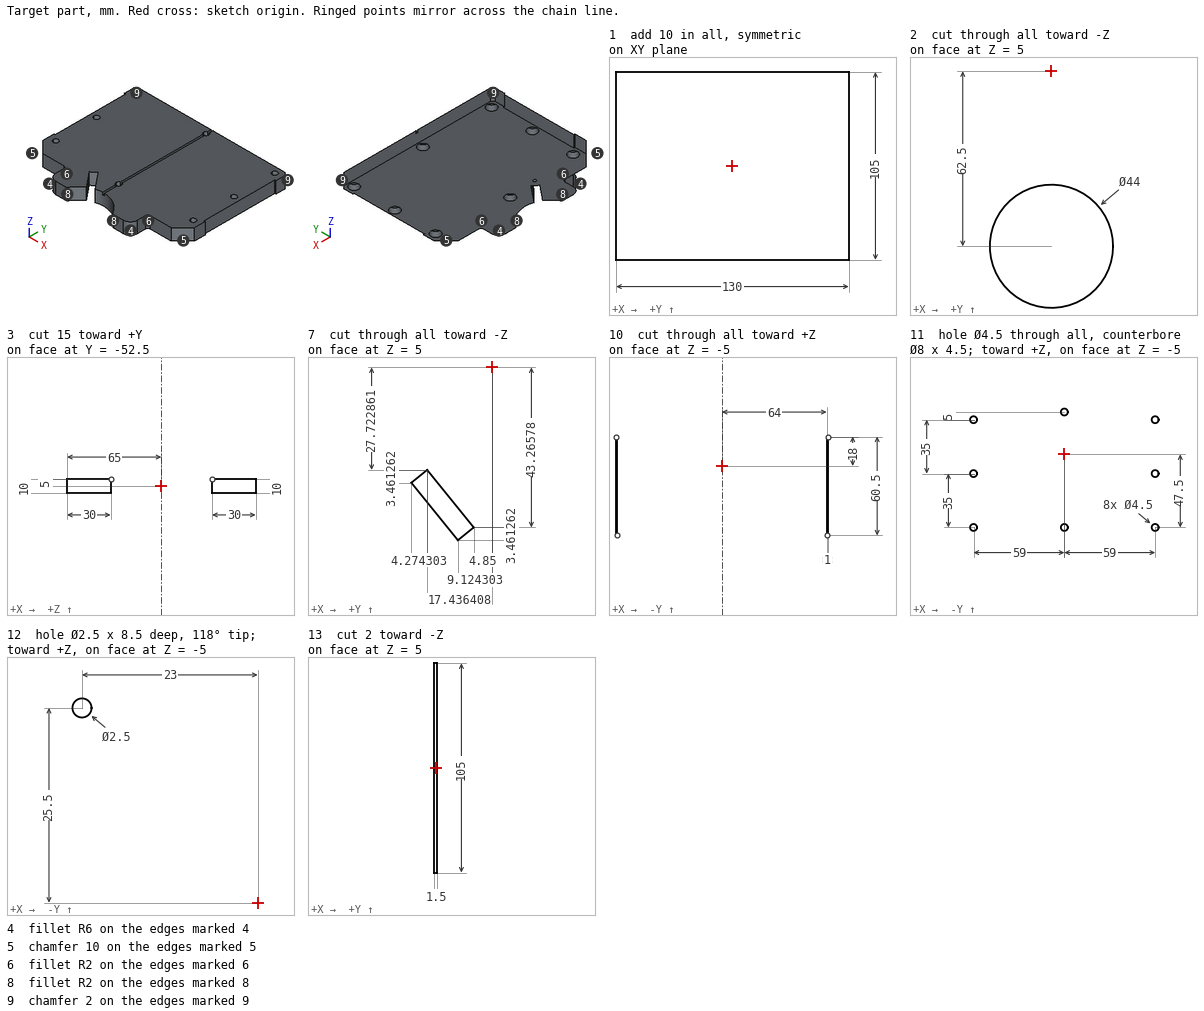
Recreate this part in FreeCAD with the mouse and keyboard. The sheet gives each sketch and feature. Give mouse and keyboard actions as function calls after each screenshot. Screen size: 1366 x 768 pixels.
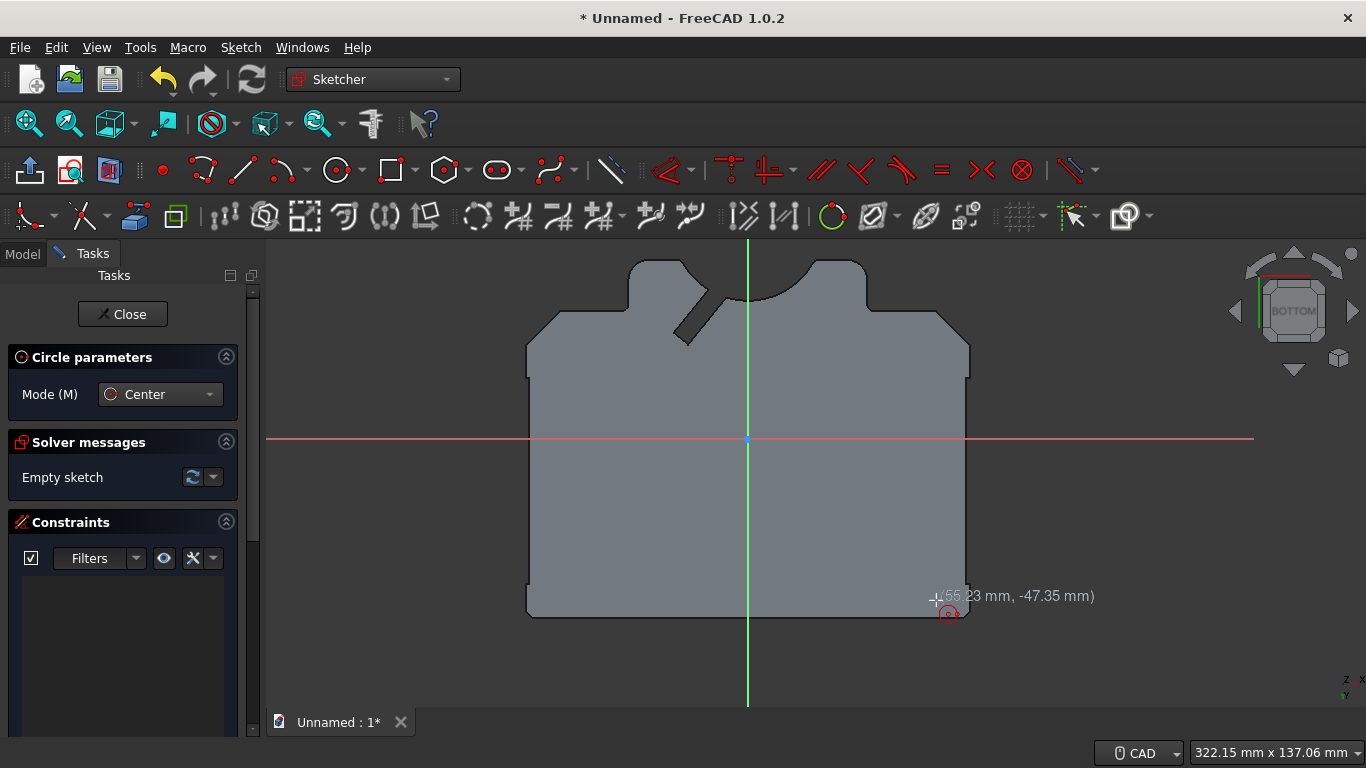
click(949, 601)
move(955, 596)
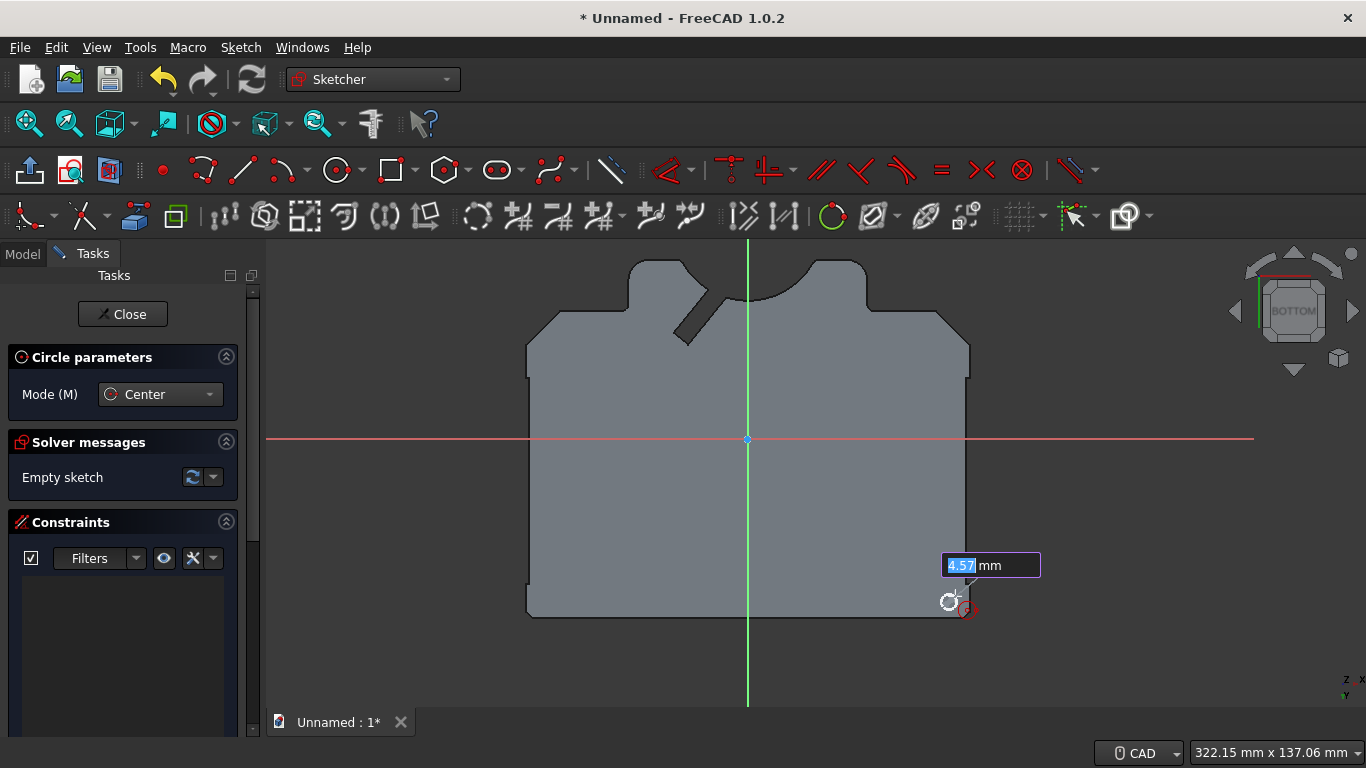
text(4.5)
key(Return)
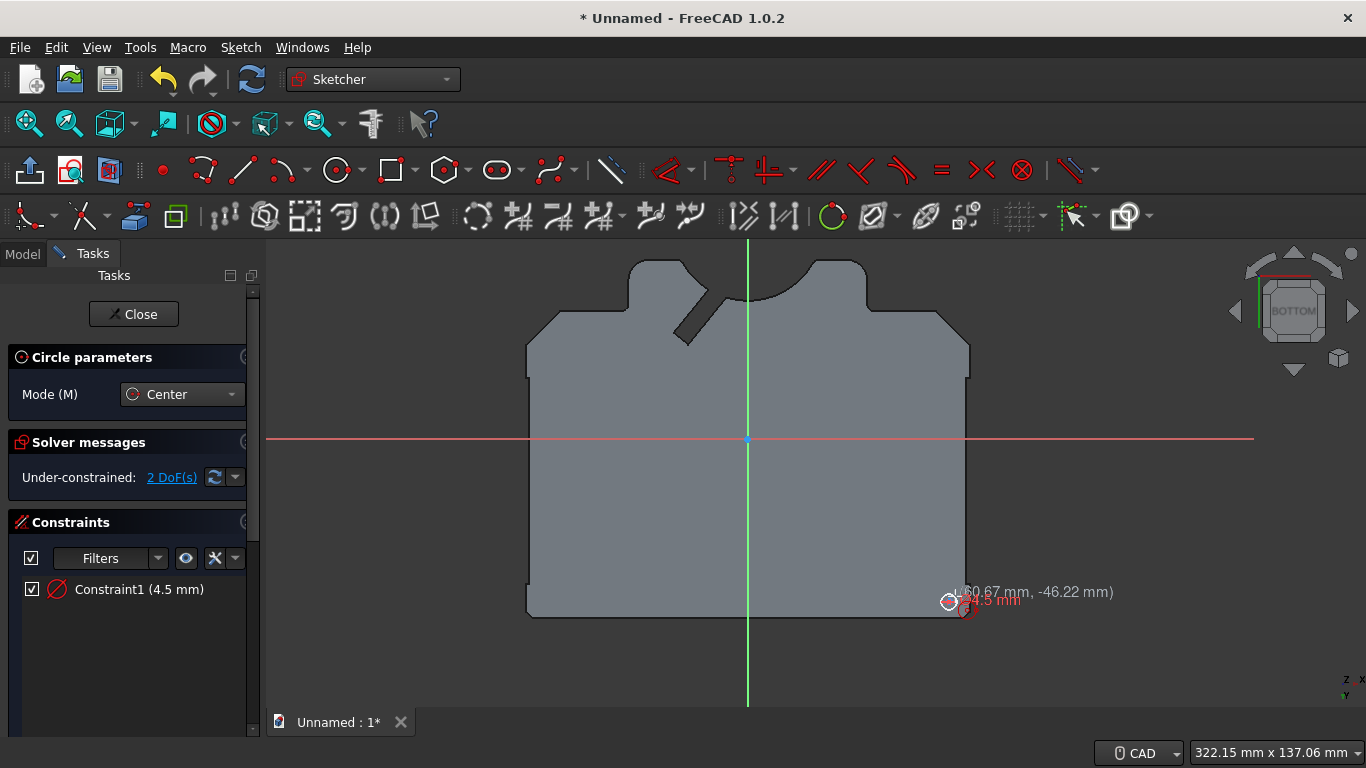
scroll(748, 601, up, 6)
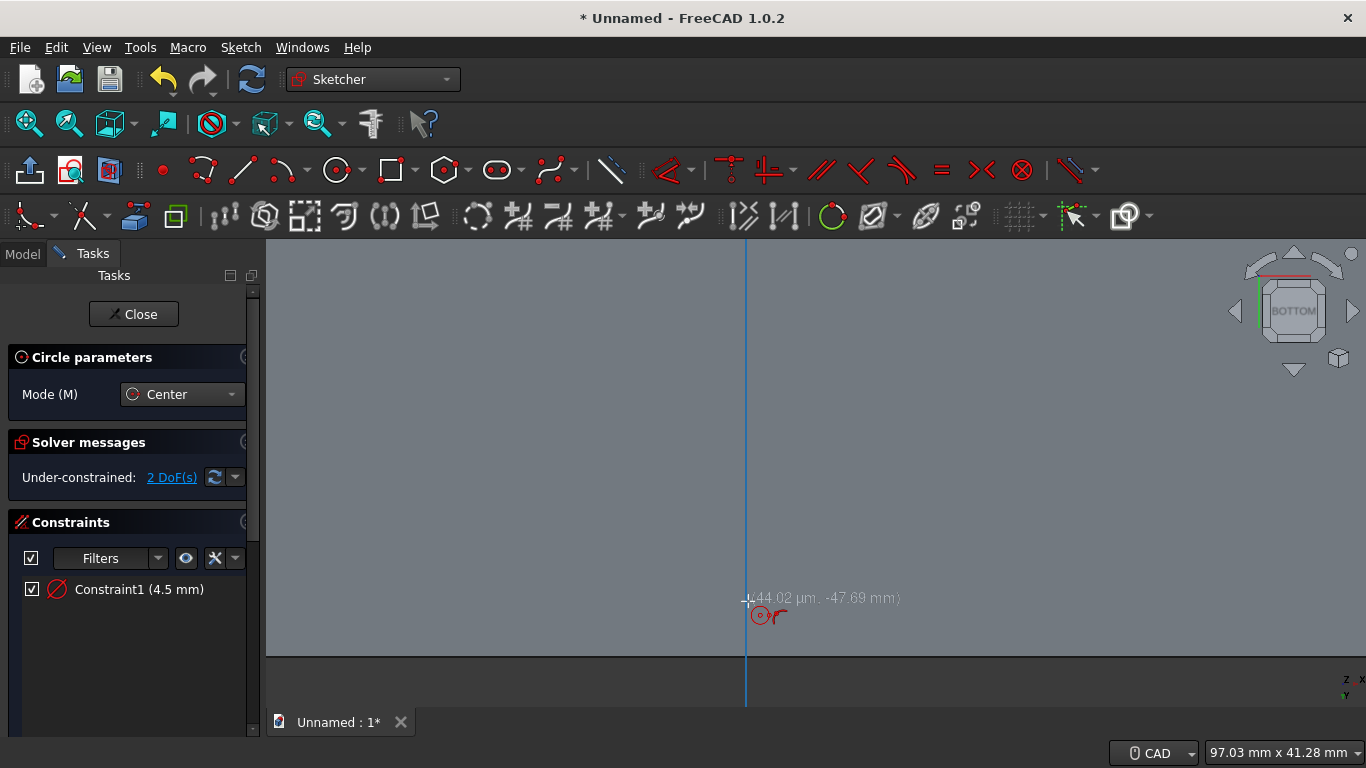
scroll(748, 601, down, 6)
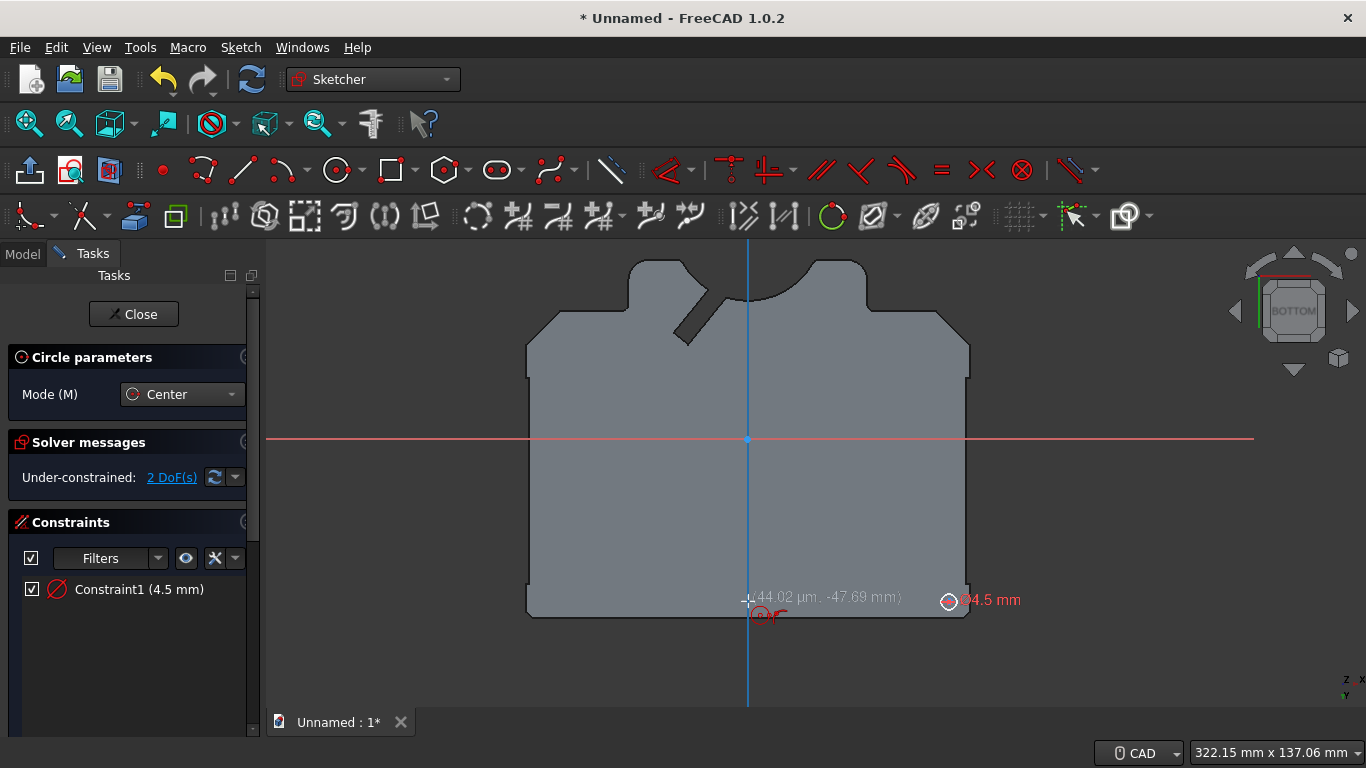
click(748, 601)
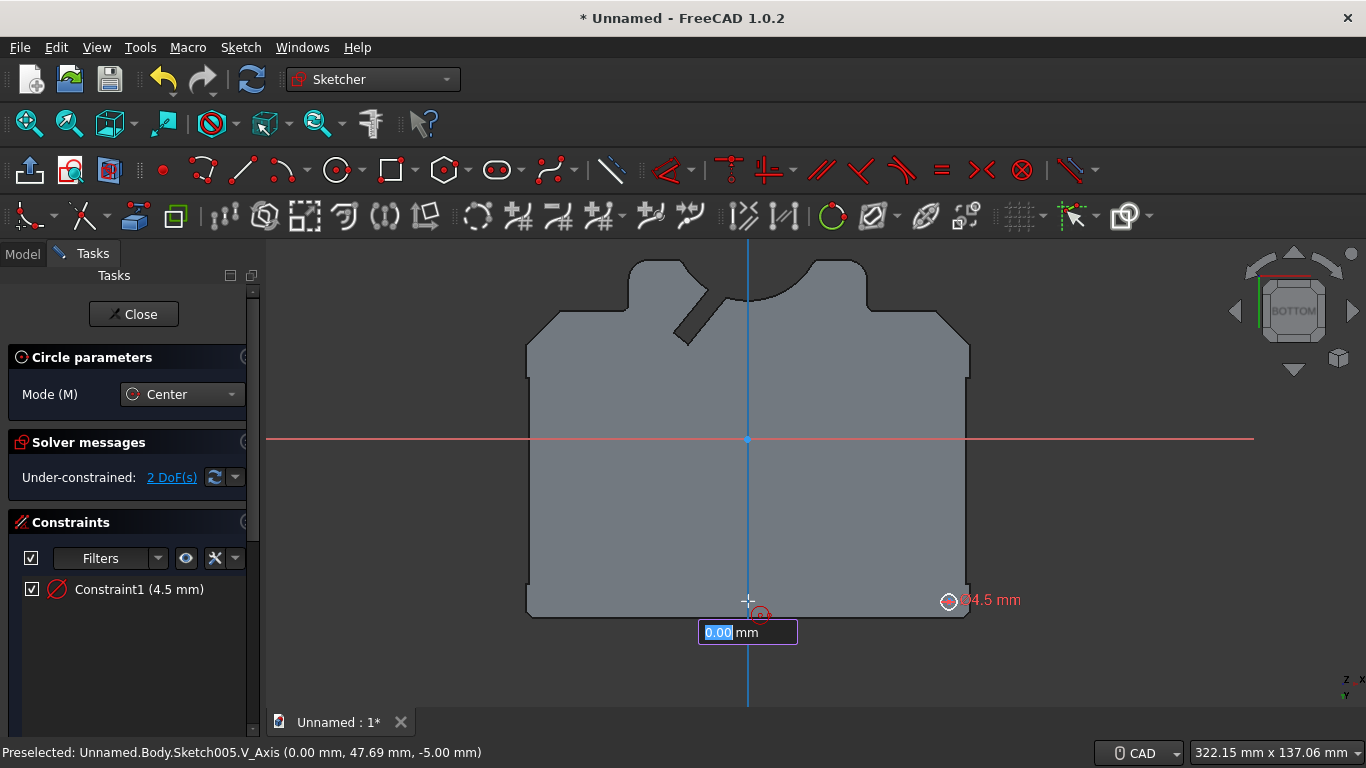
scroll(755, 599, up, 4)
move(755, 597)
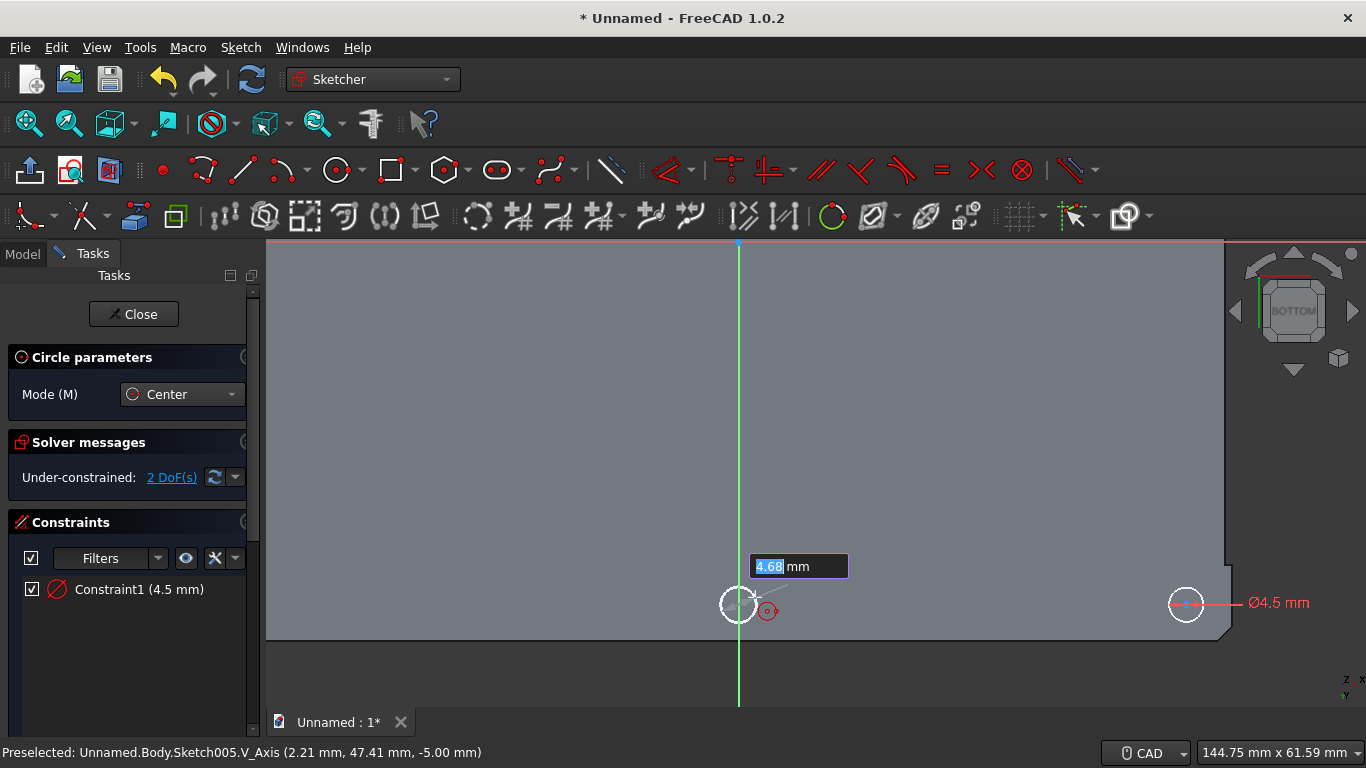
text(4.5)
key(Return)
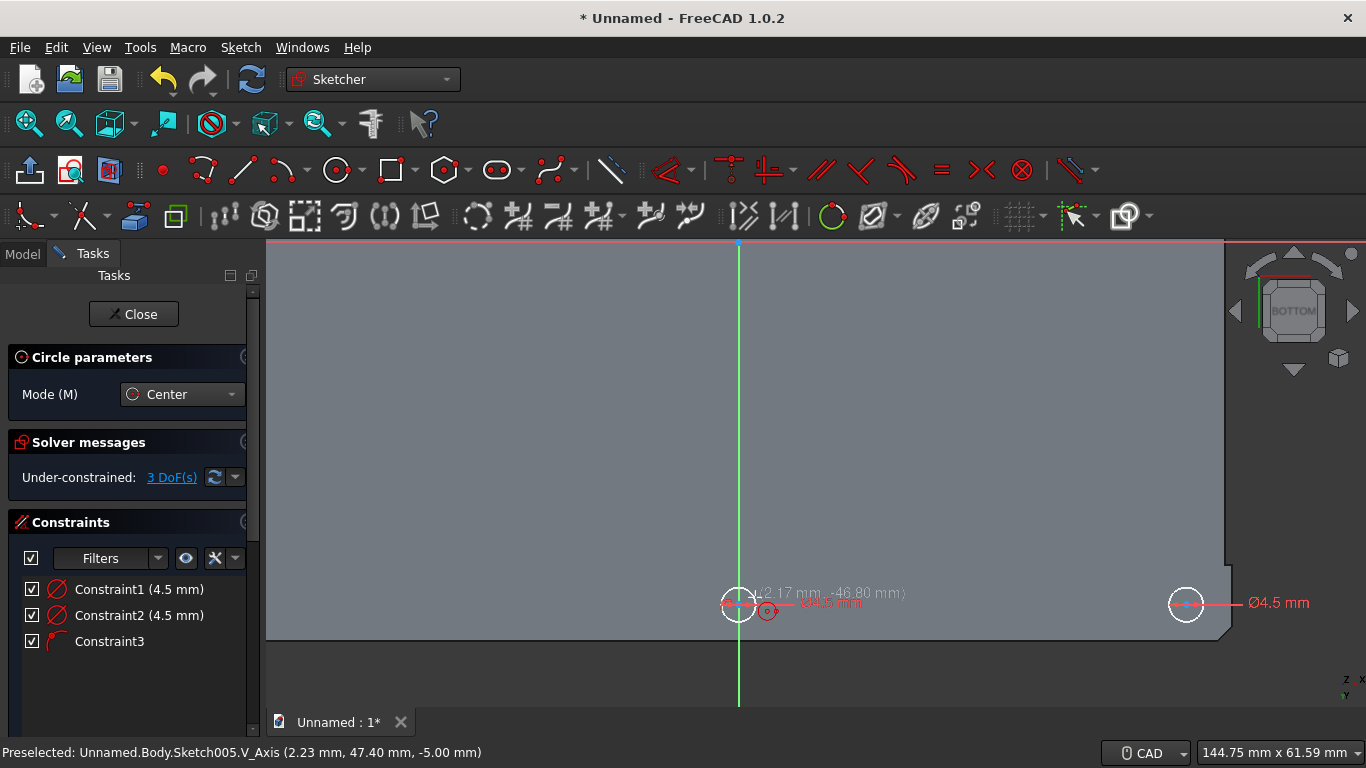
scroll(755, 599, down, 4)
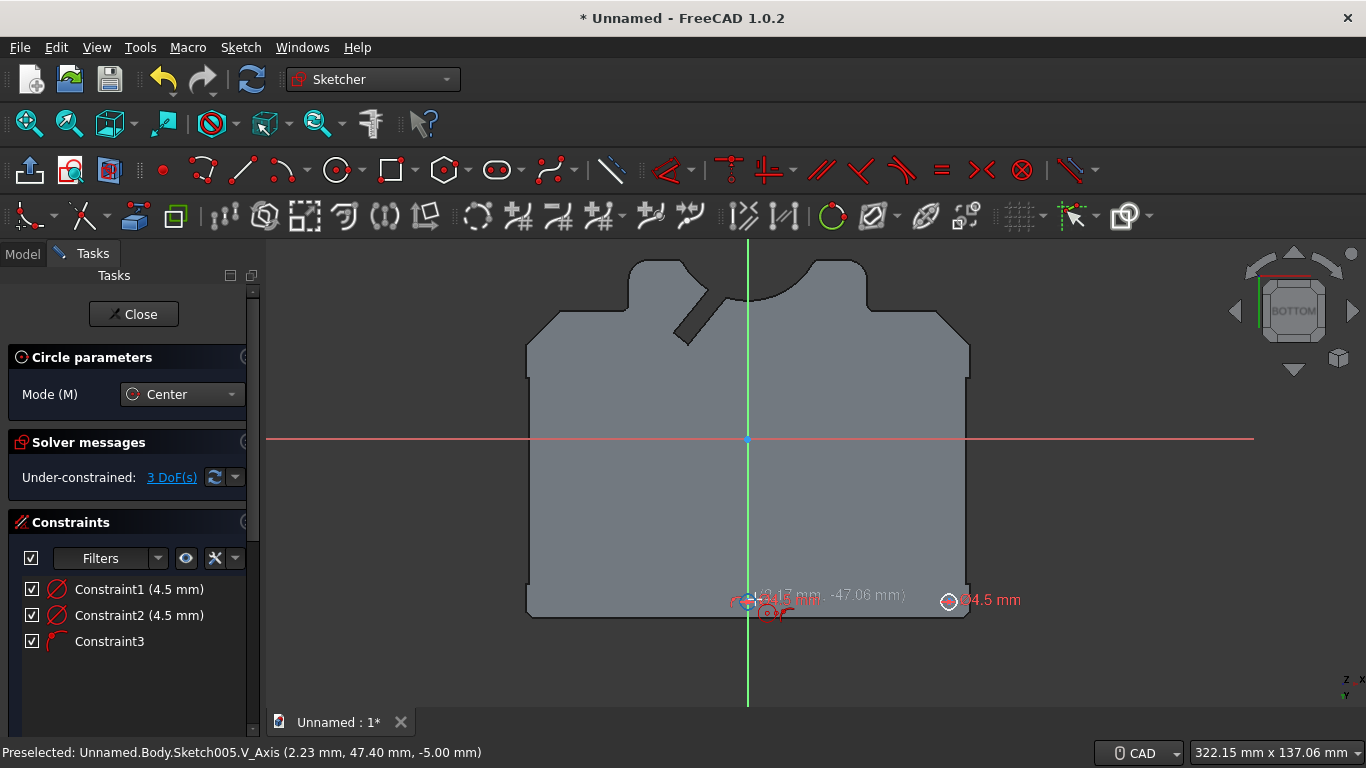
scroll(546, 601, up, 6)